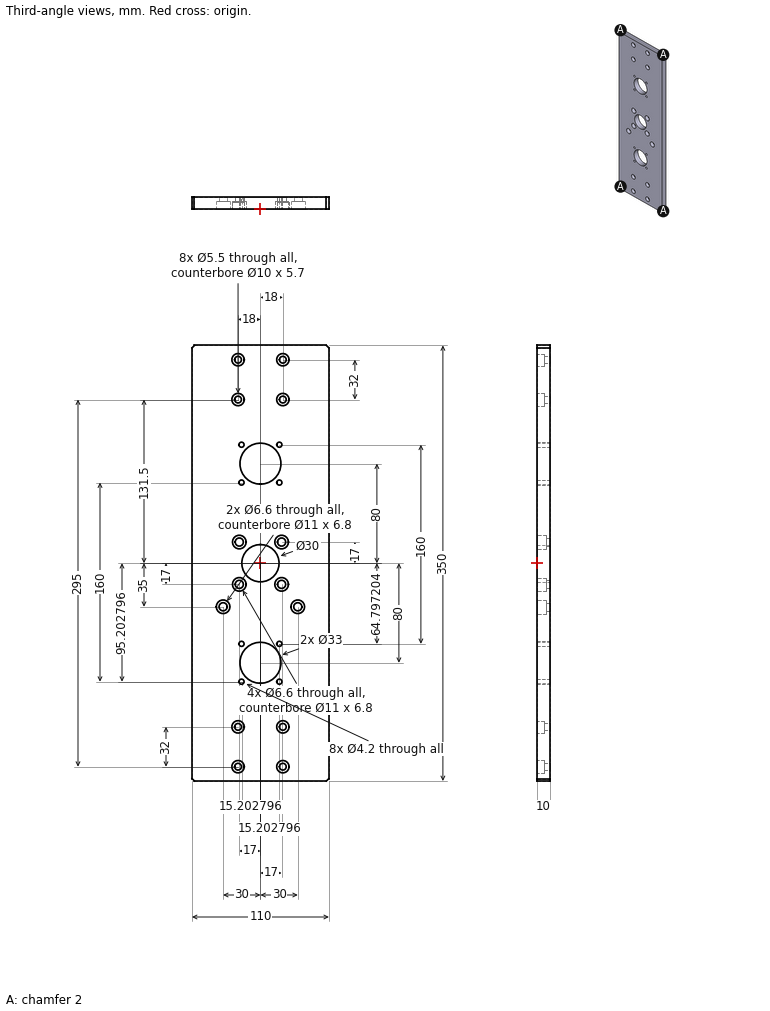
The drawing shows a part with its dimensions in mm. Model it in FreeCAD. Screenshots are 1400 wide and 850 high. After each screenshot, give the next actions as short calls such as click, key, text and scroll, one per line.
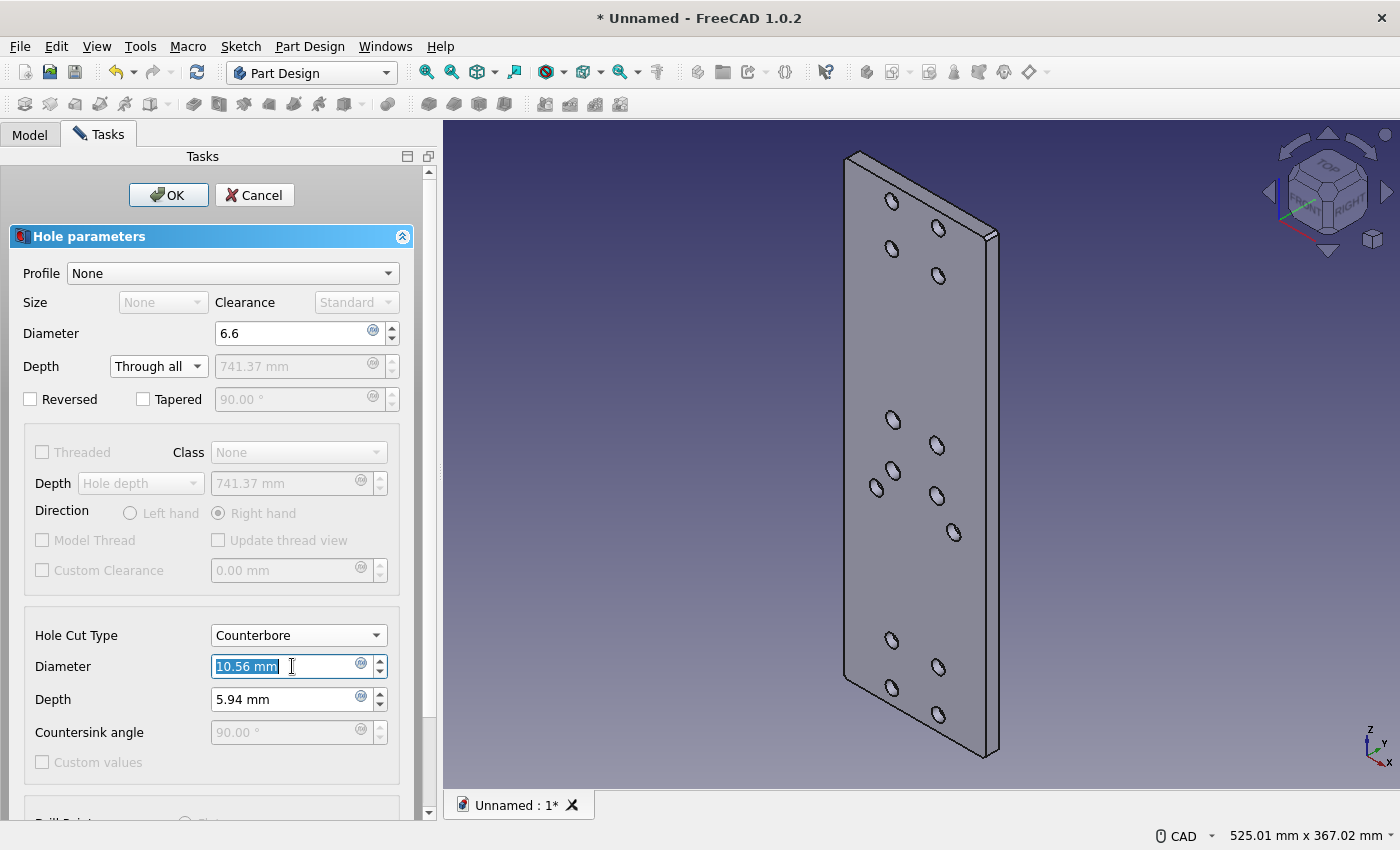
text(11)
key(Tab)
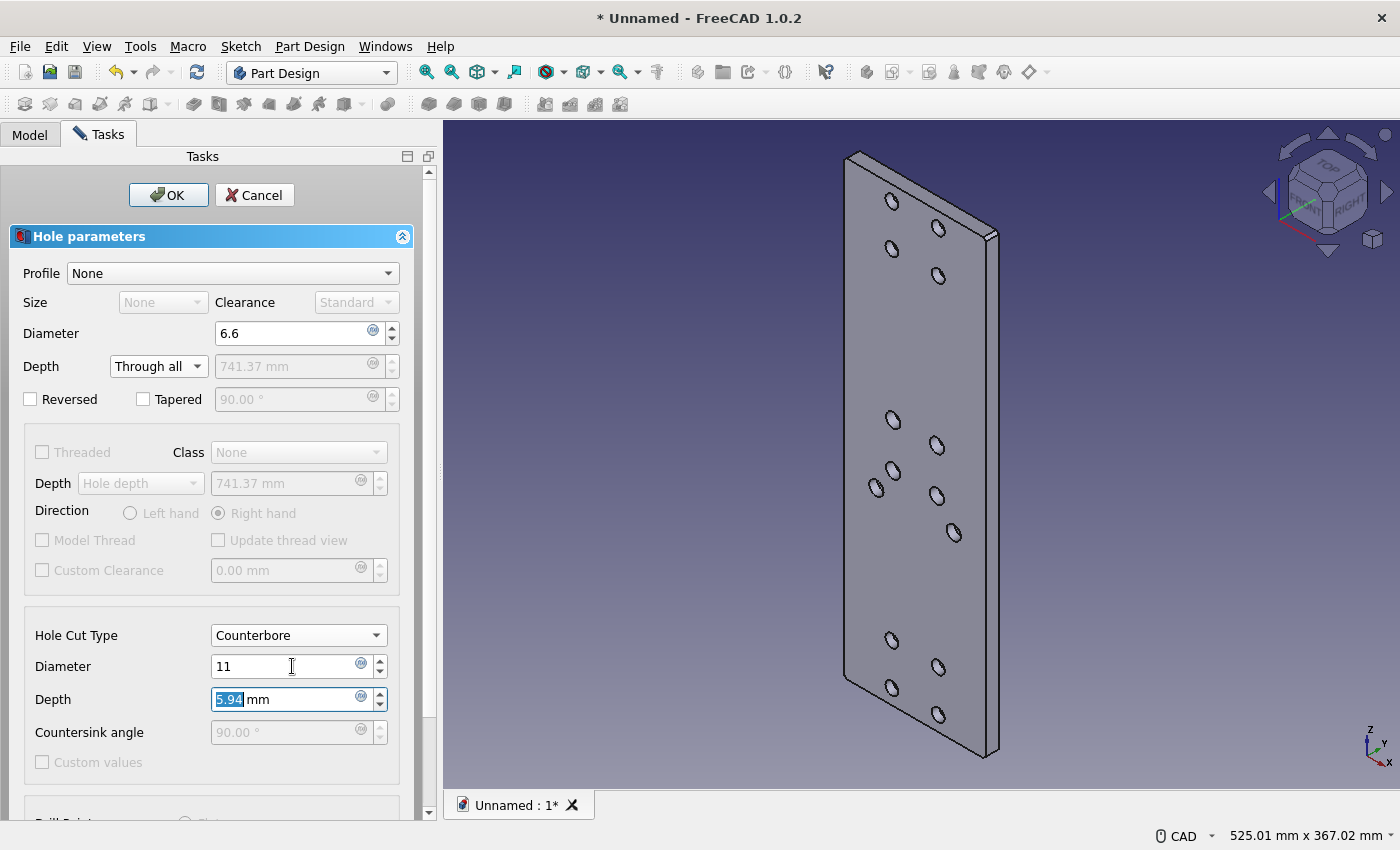
text(6.8)
key(Tab)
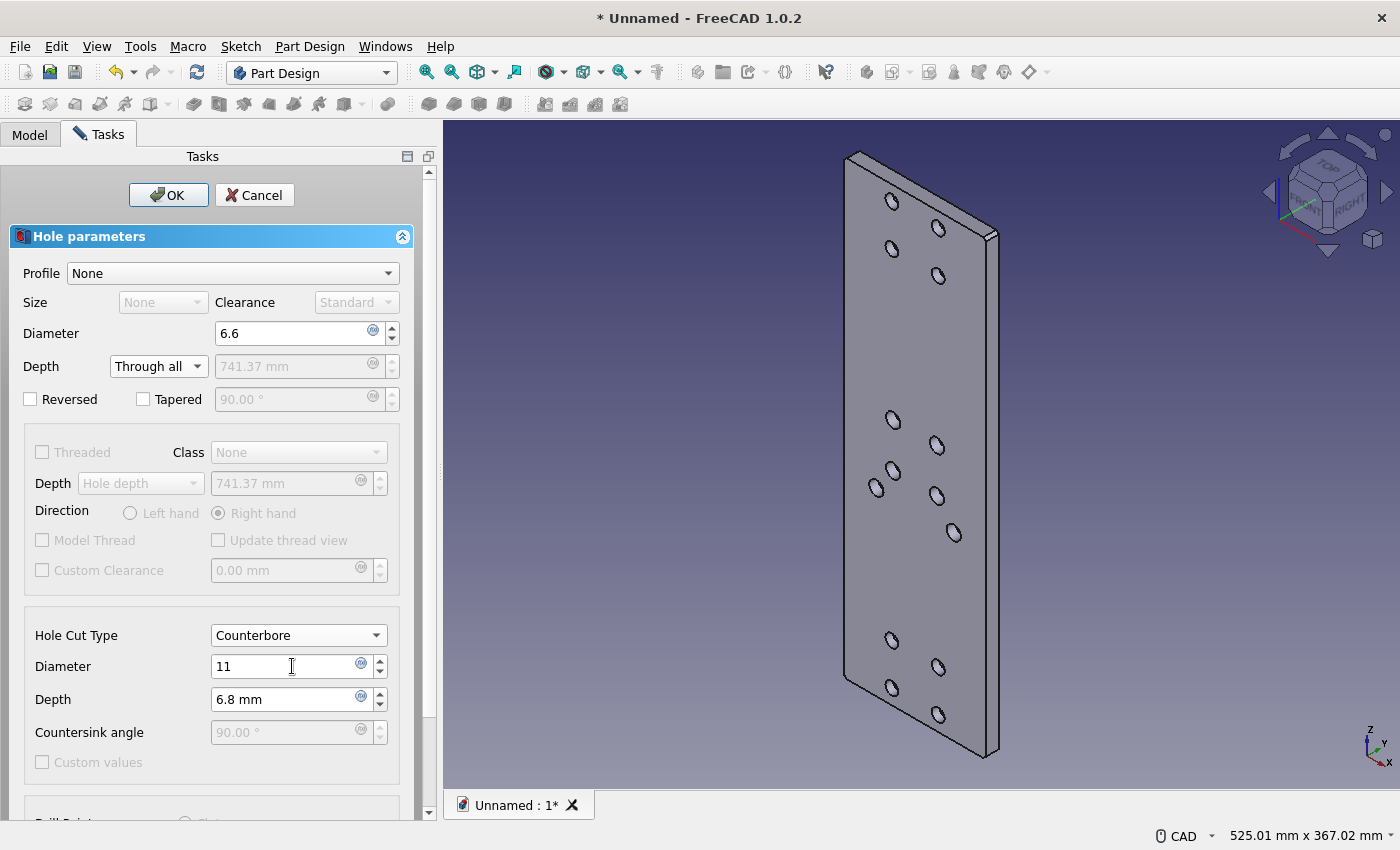
click(169, 195)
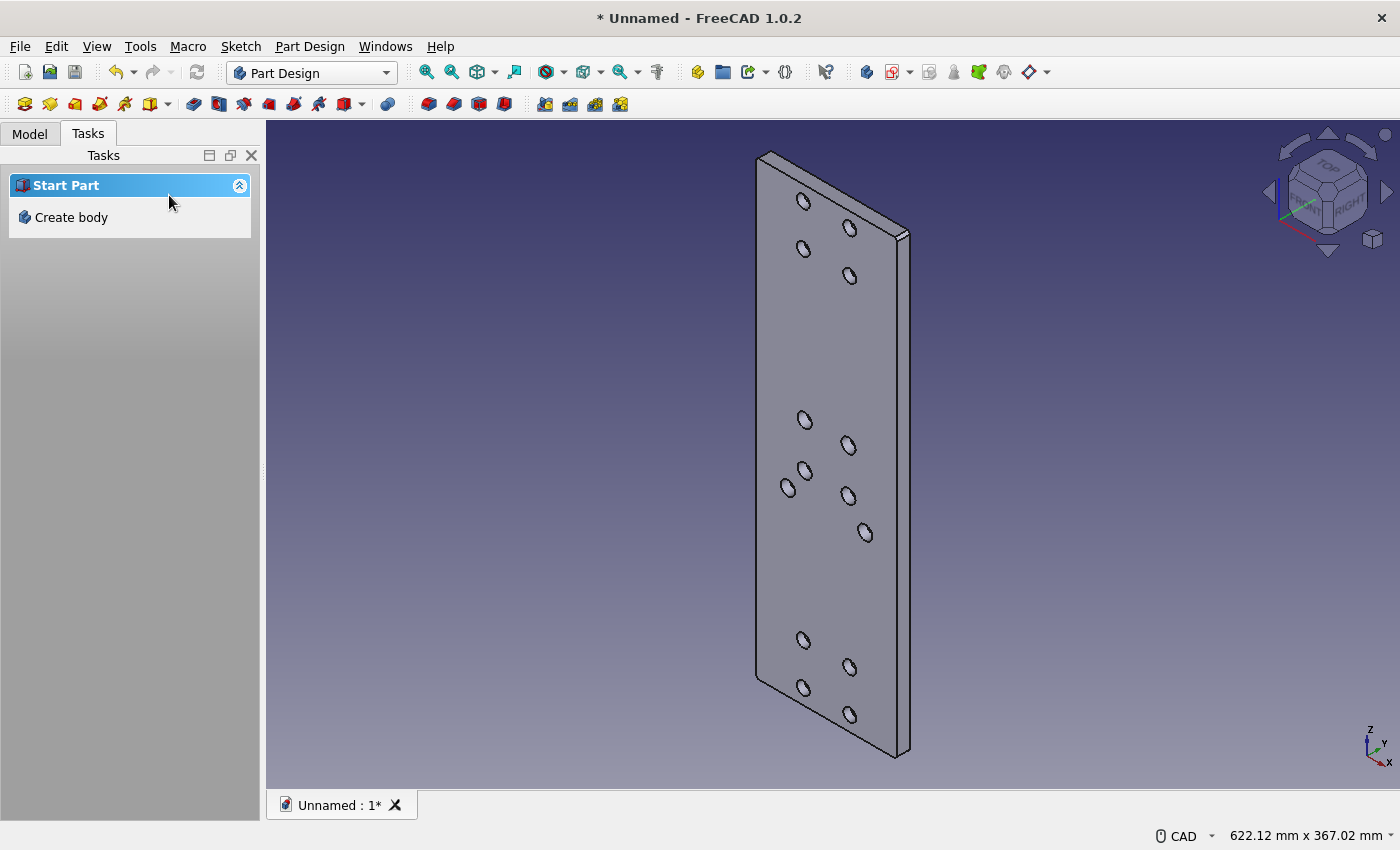
click(892, 72)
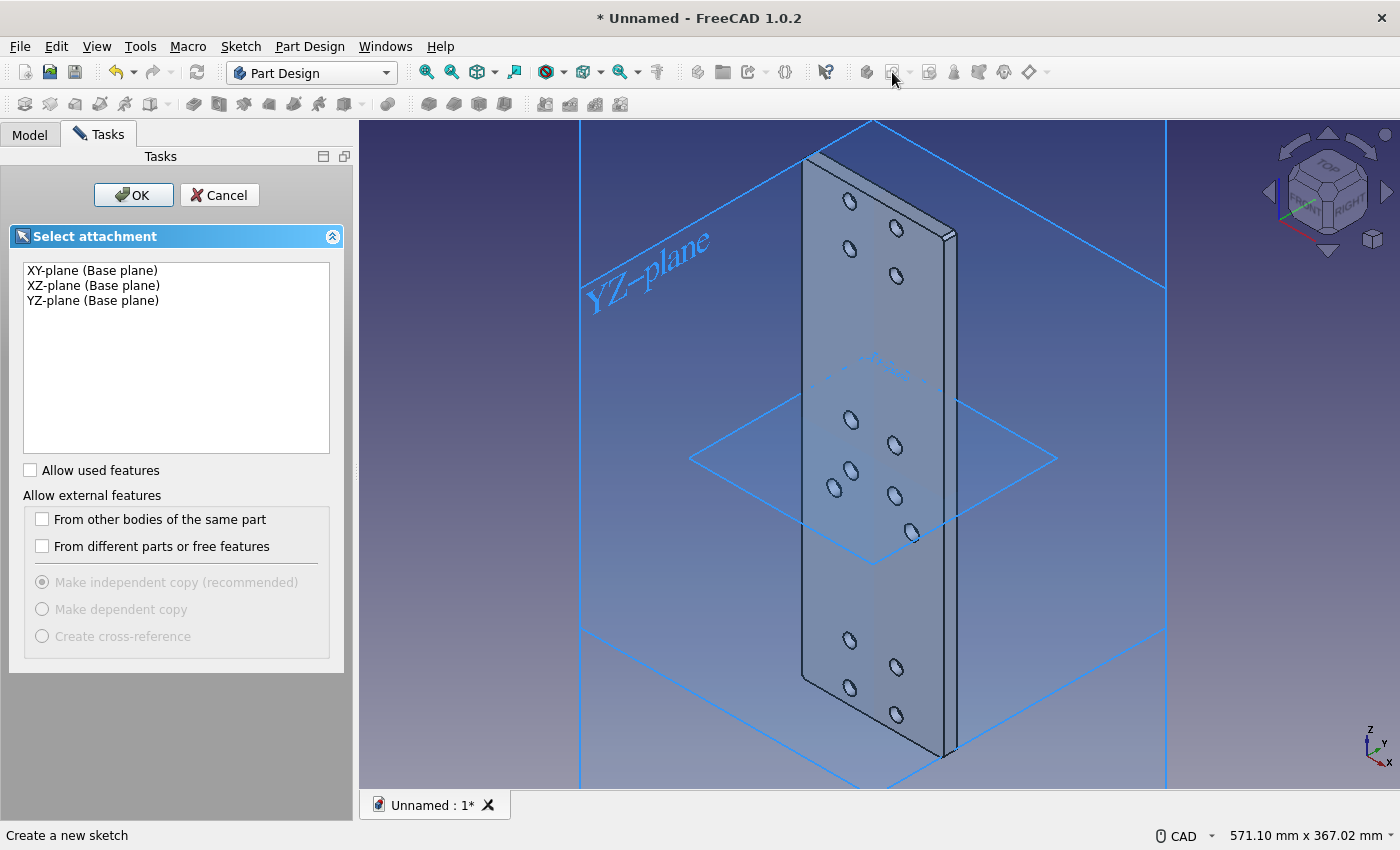
click(84, 286)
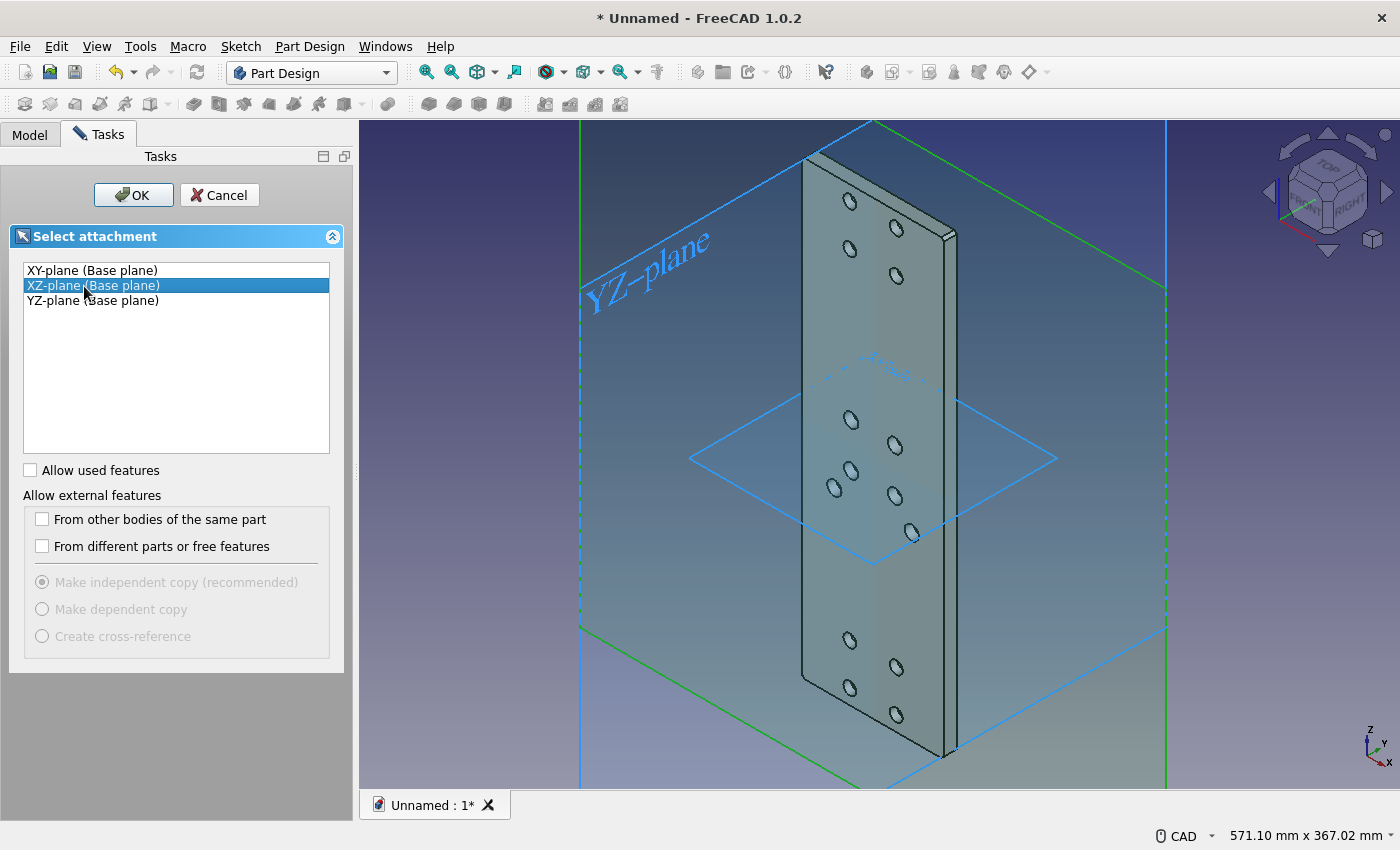
click(134, 195)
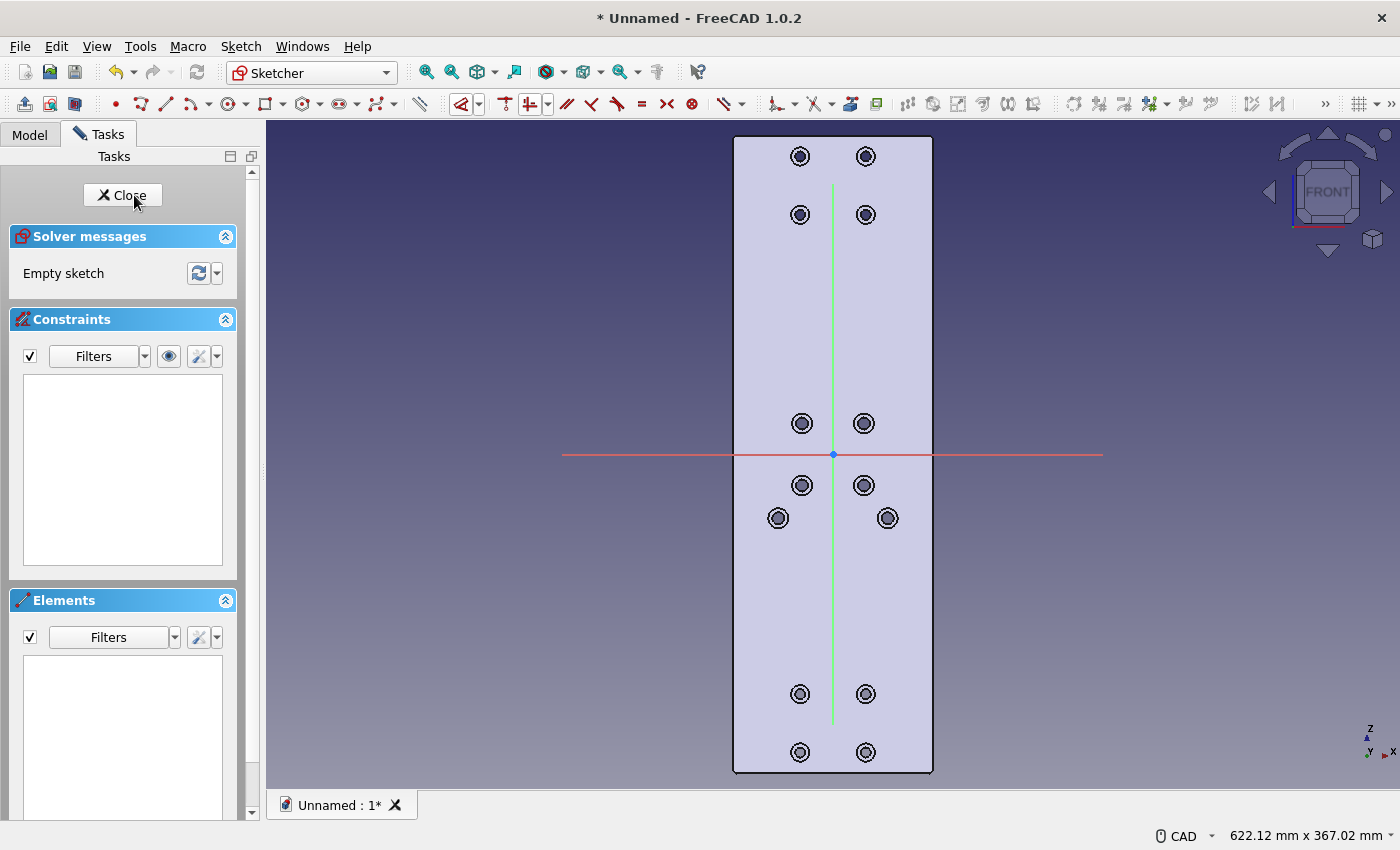
click(228, 104)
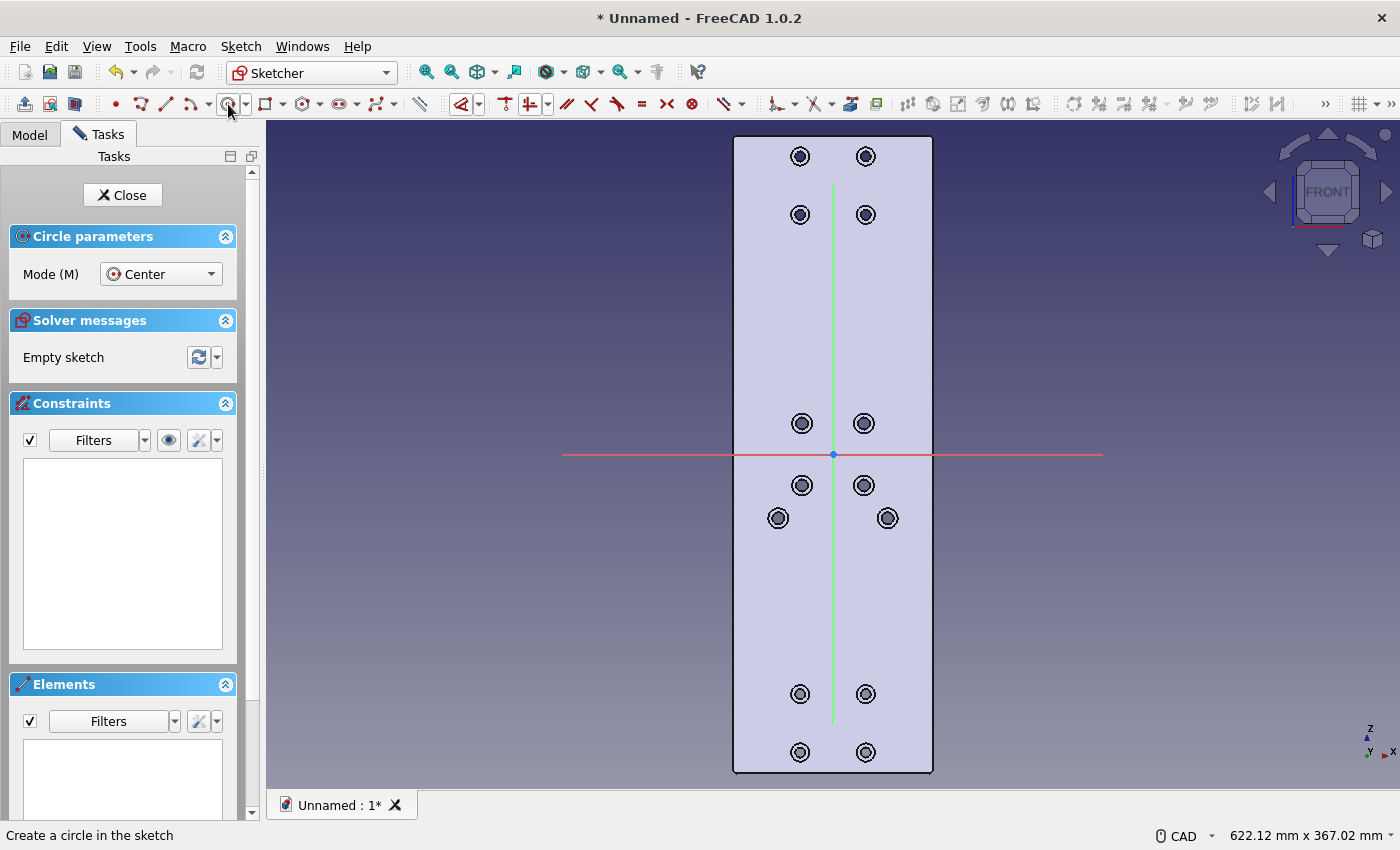
click(833, 600)
move(854, 579)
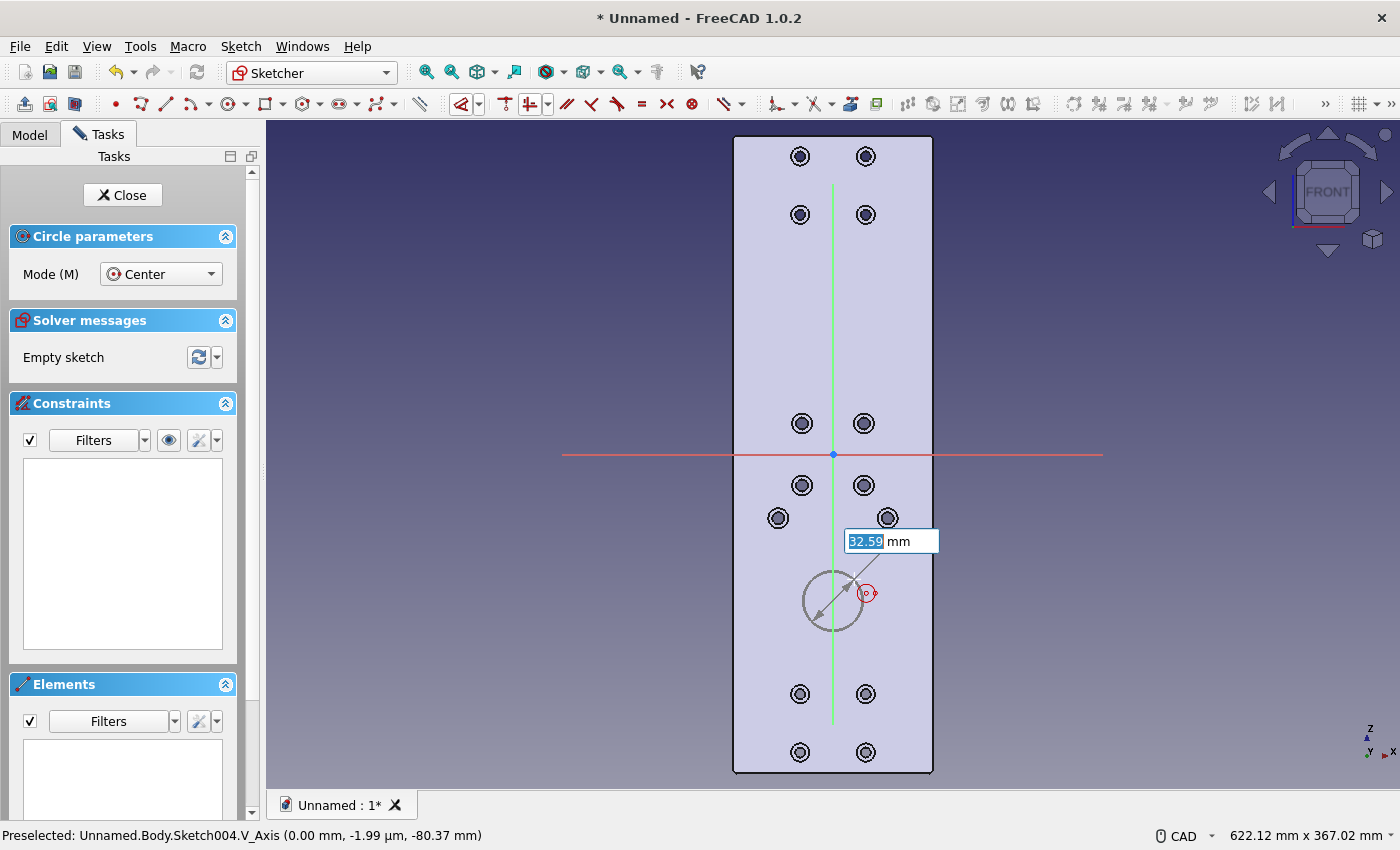
text(33)
key(Return)